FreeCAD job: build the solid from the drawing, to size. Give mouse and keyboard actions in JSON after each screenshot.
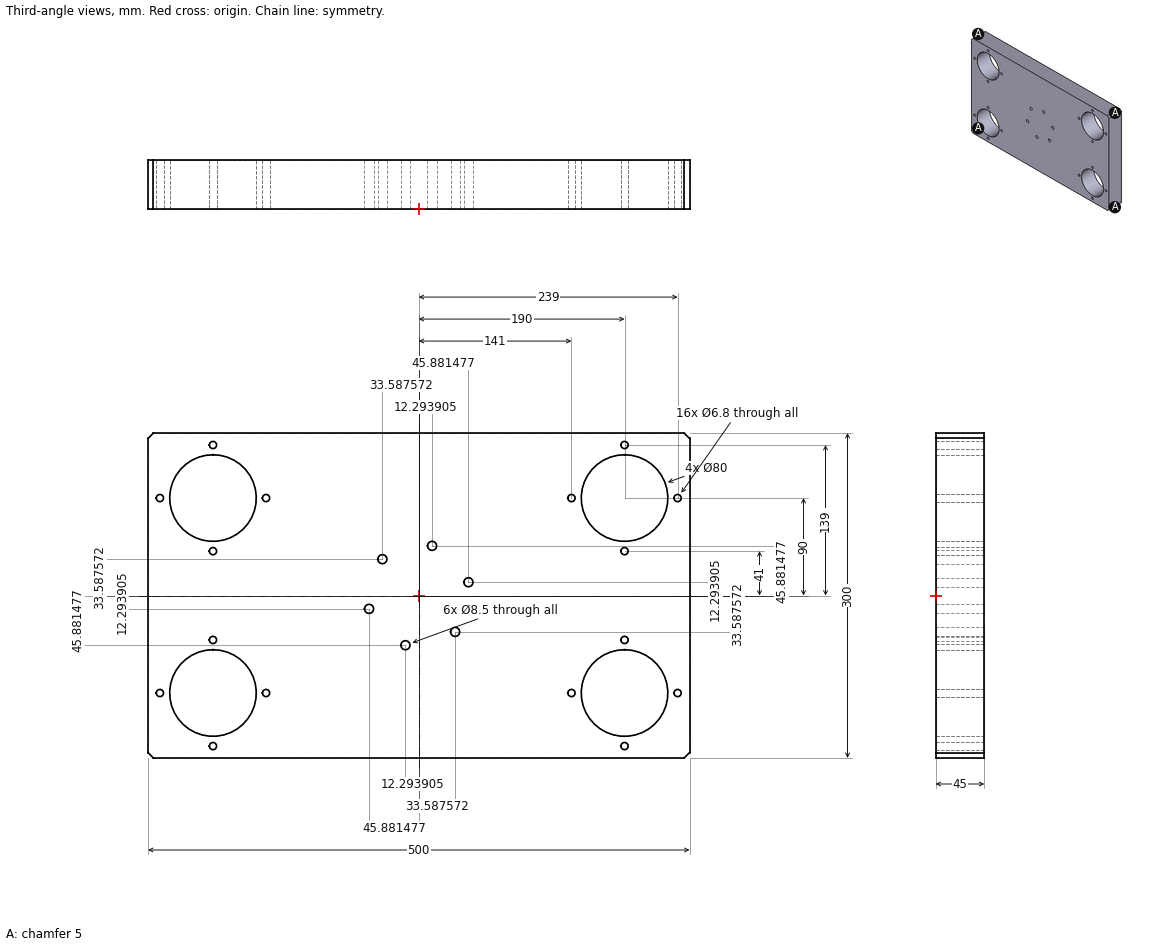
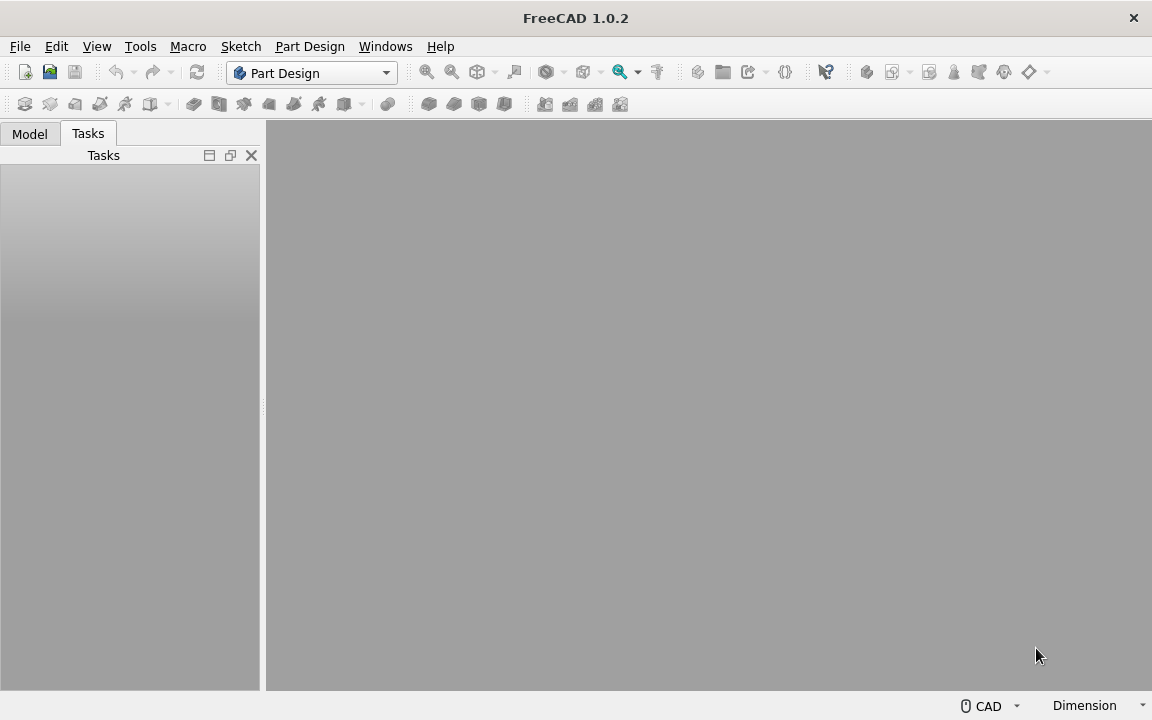
{"action": "left_click", "coordinate": [25, 72]}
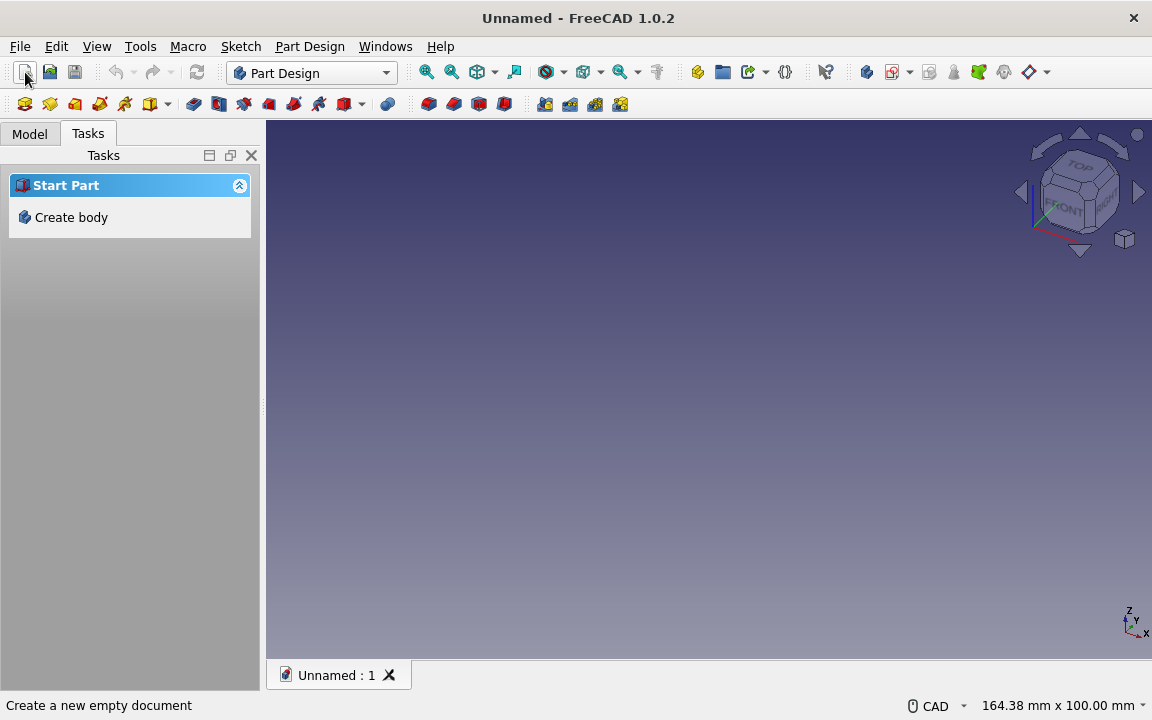
{"action": "left_click", "coordinate": [892, 72]}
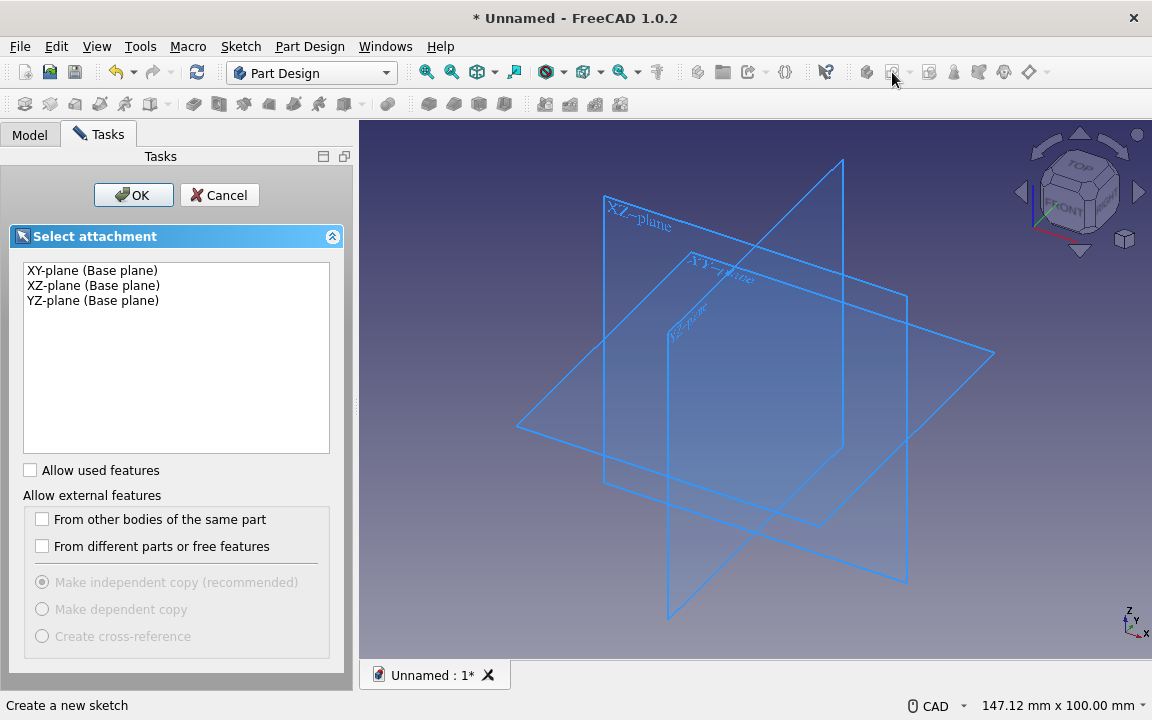
{"action": "left_click", "coordinate": [84, 286]}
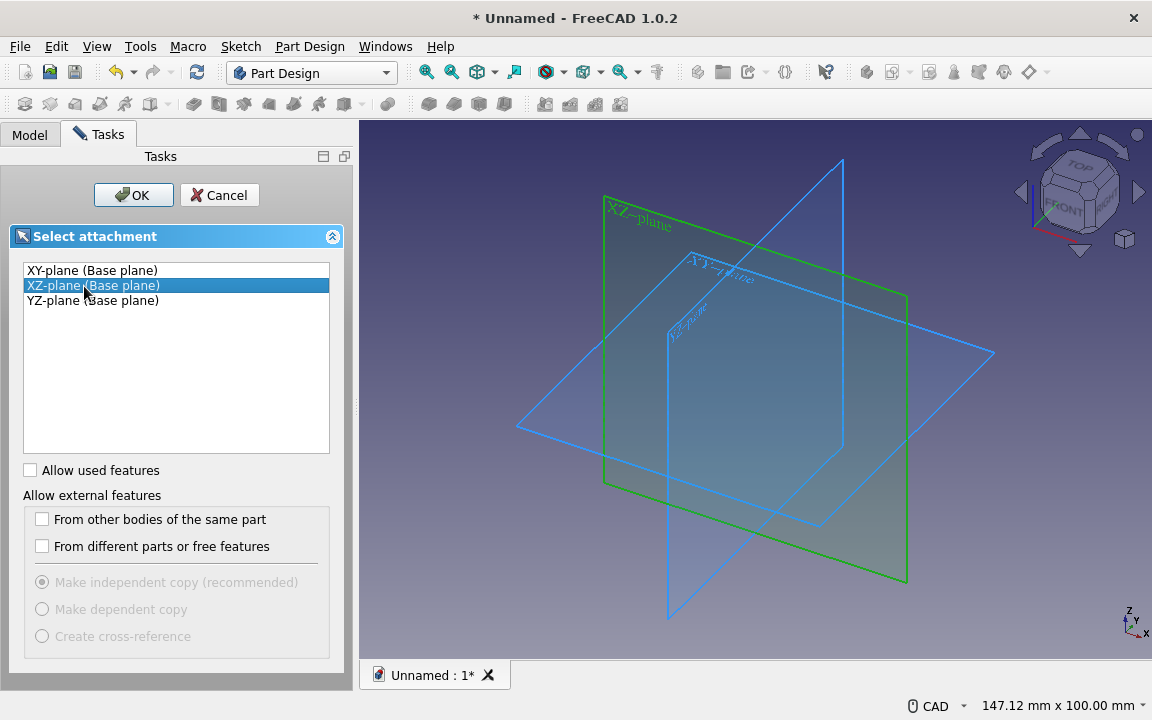
{"action": "left_click", "coordinate": [134, 195]}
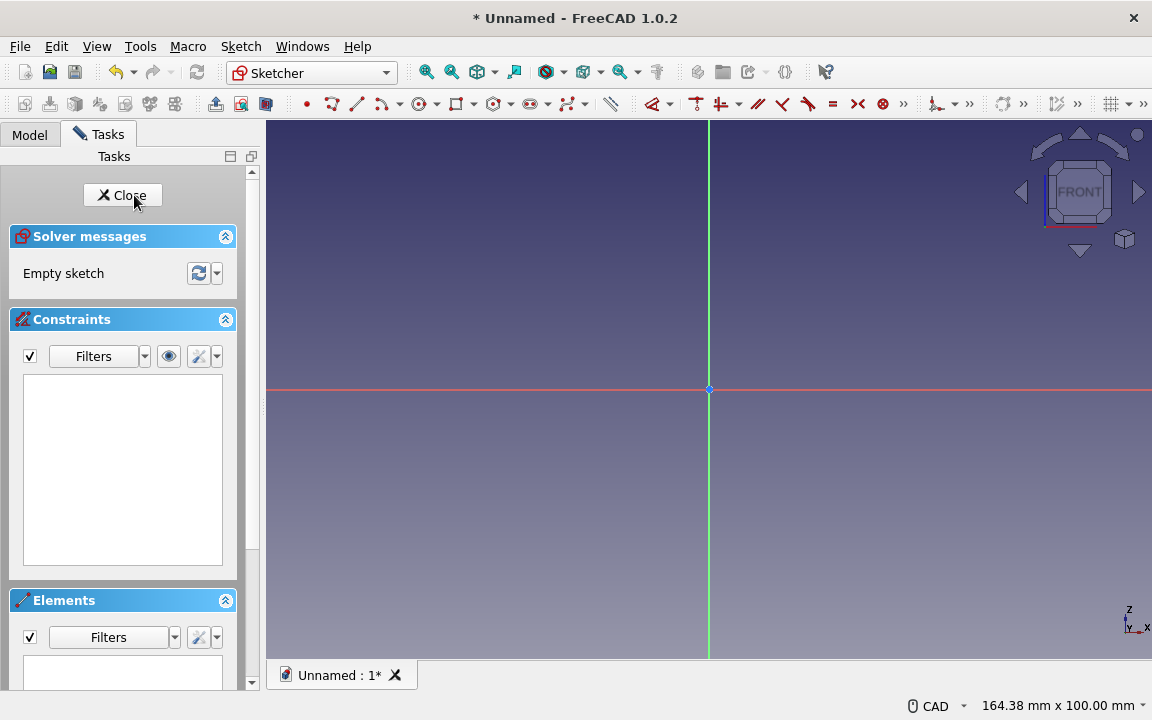
{"action": "scroll", "coordinate": [627, 390], "scroll_direction": "down", "scroll_amount": 9}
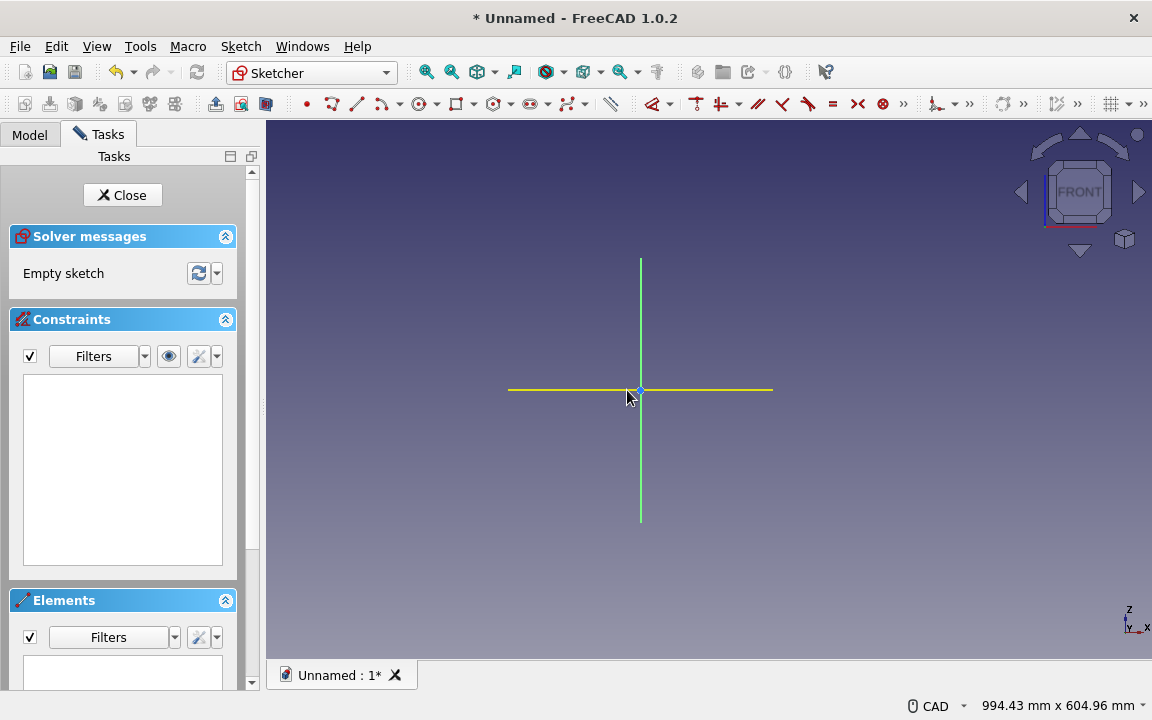
{"action": "key", "text": "g v"}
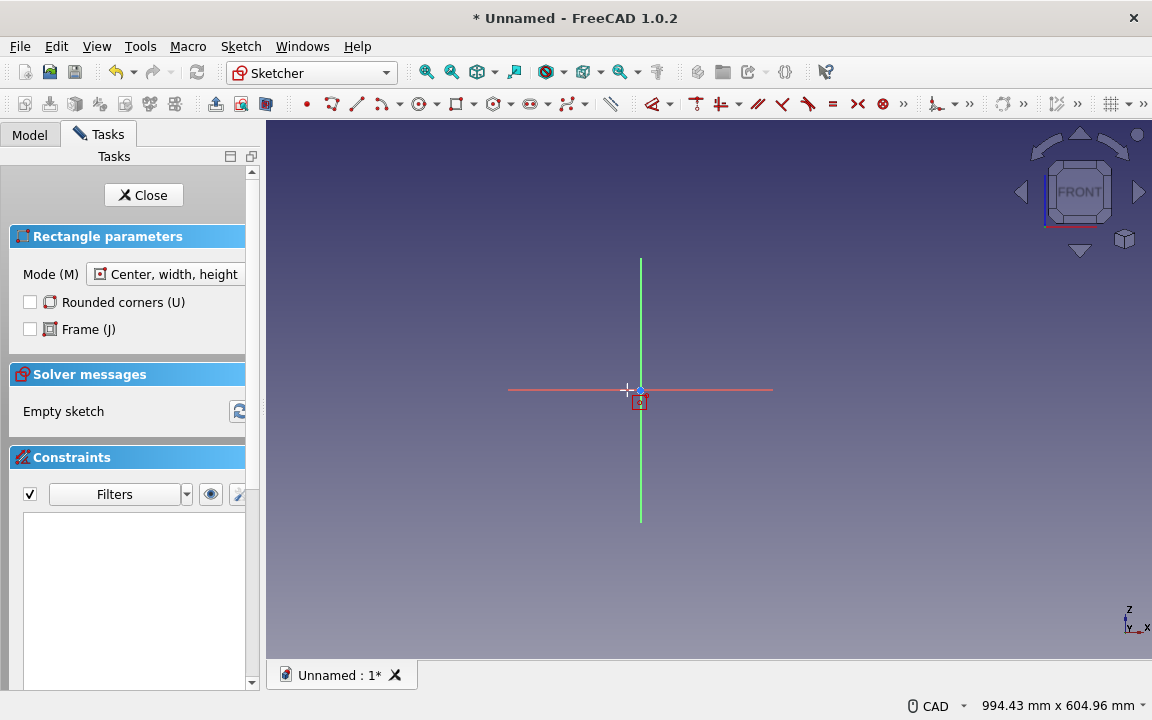
{"action": "left_click", "coordinate": [641, 390]}
{"action": "left_click", "coordinate": [864, 257]}
{"action": "key", "text": "Escape"}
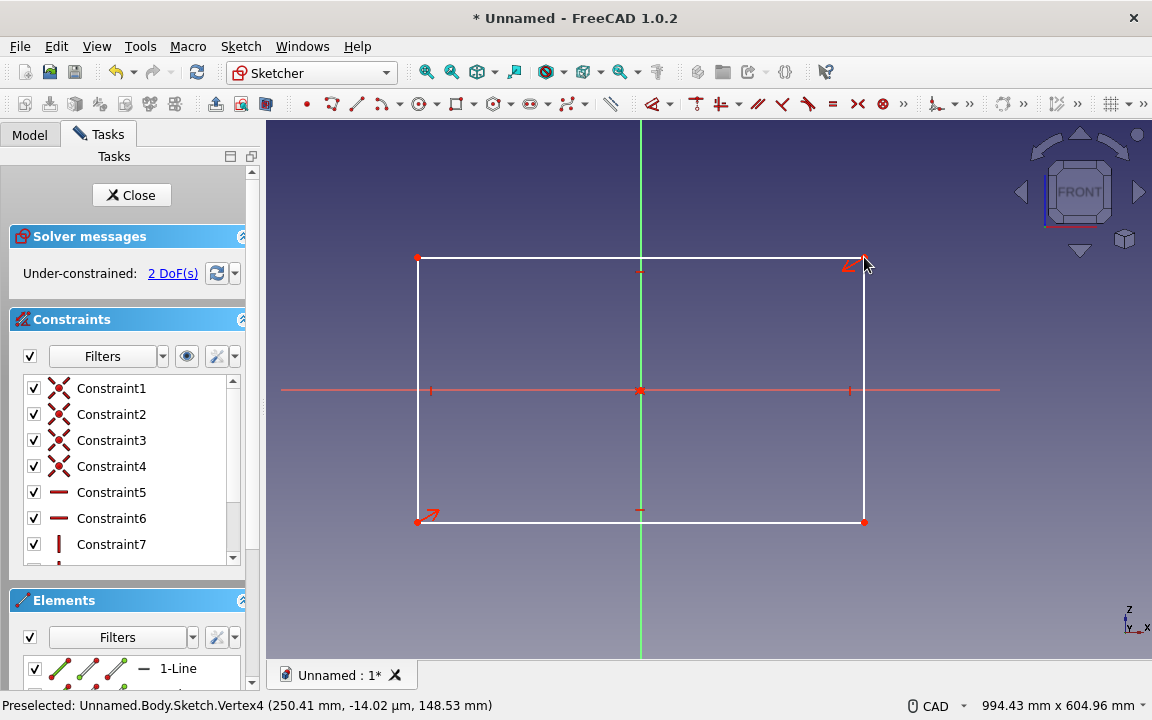
{"action": "left_click", "coordinate": [652, 104]}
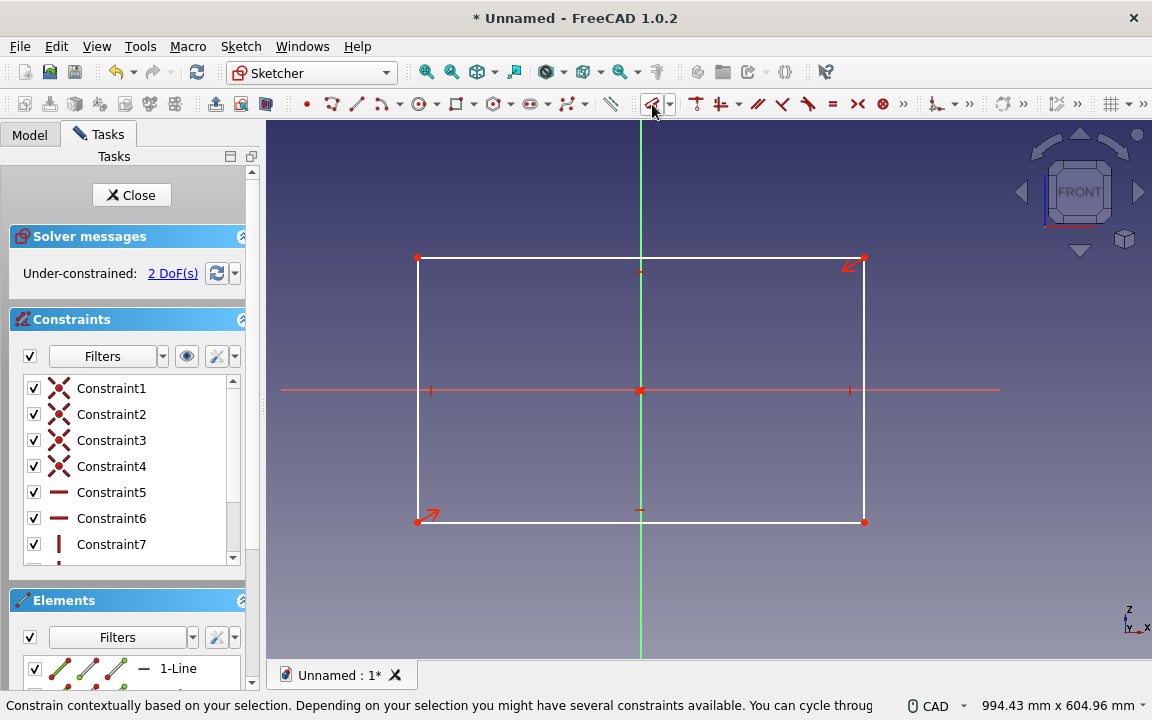
{"action": "left_click", "coordinate": [552, 523]}
{"action": "left_click", "coordinate": [538, 557]}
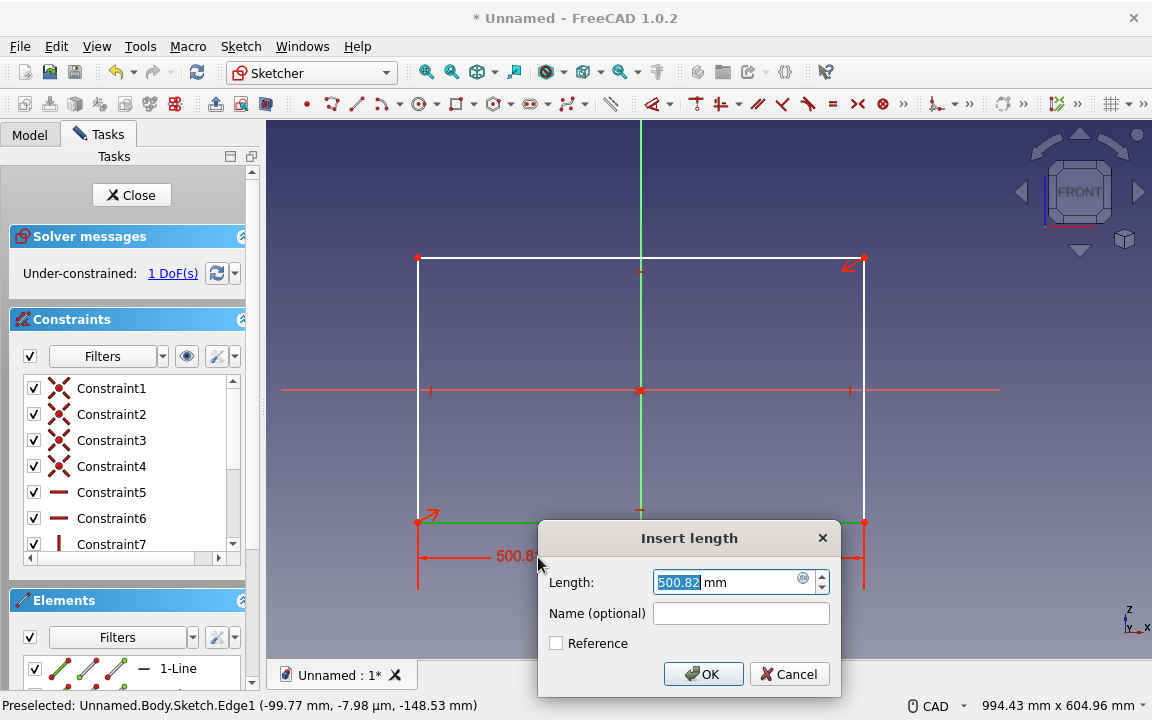
{"action": "type", "text": "500"}
{"action": "key", "text": "Return"}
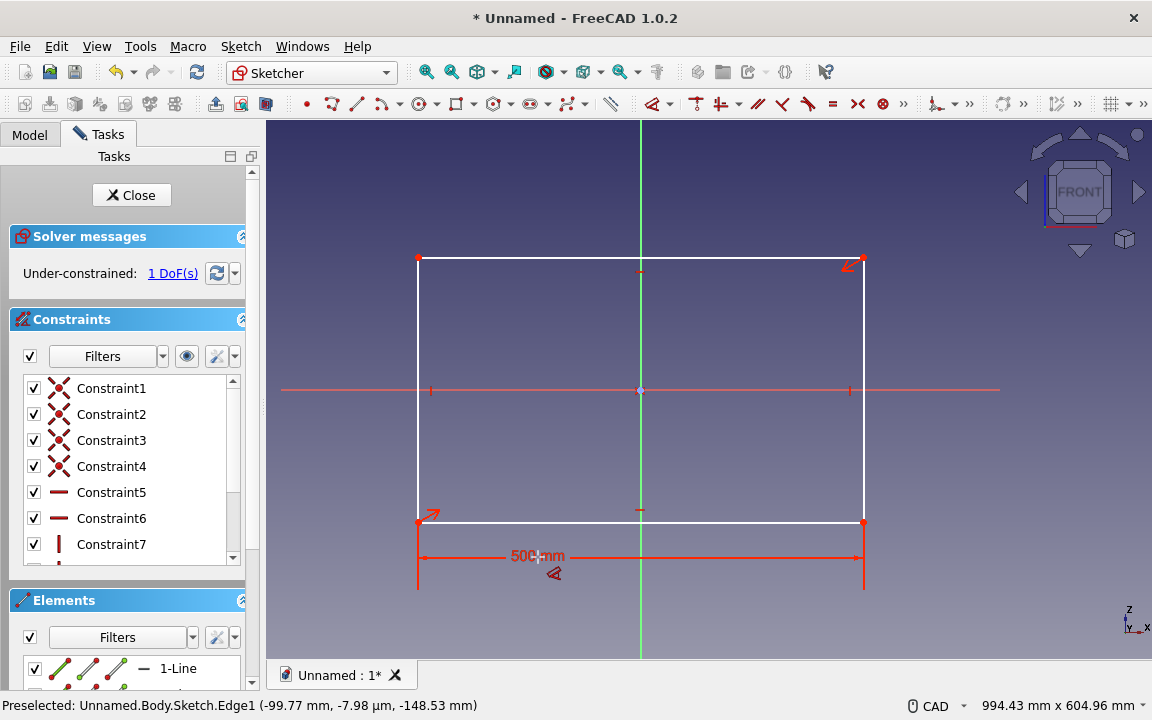
{"action": "left_click", "coordinate": [864, 443]}
{"action": "left_click", "coordinate": [898, 329]}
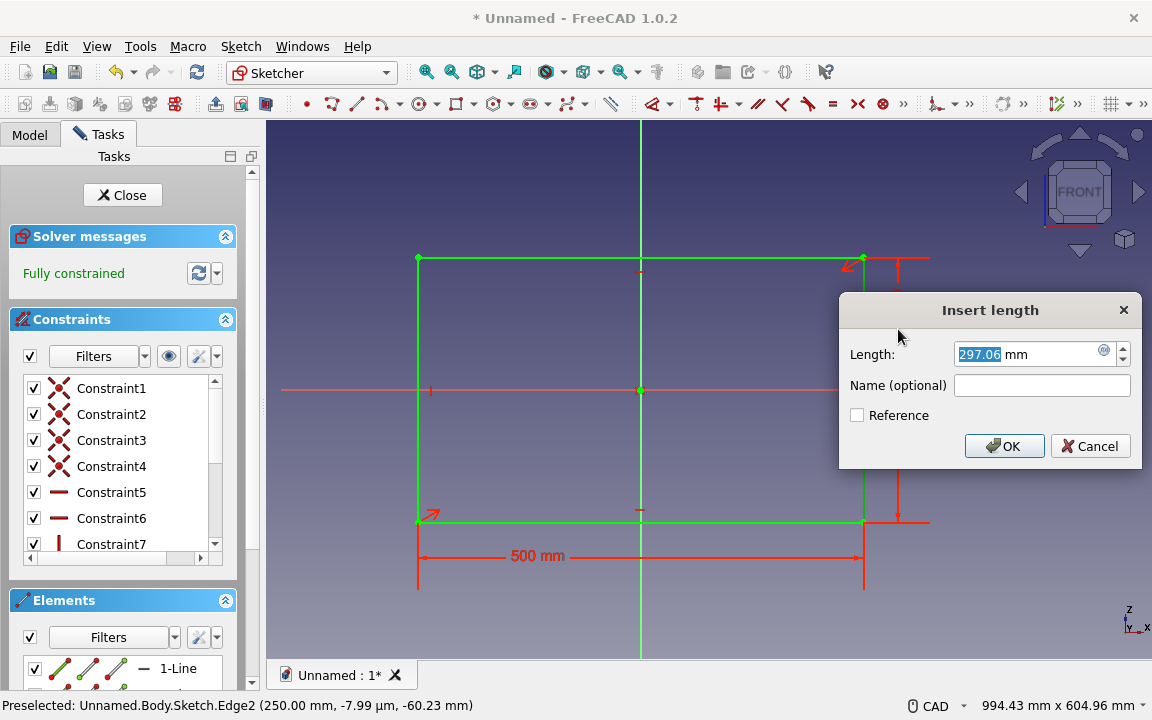
{"action": "type", "text": "300"}
{"action": "key", "text": "Return"}
{"action": "key", "text": "Escape"}